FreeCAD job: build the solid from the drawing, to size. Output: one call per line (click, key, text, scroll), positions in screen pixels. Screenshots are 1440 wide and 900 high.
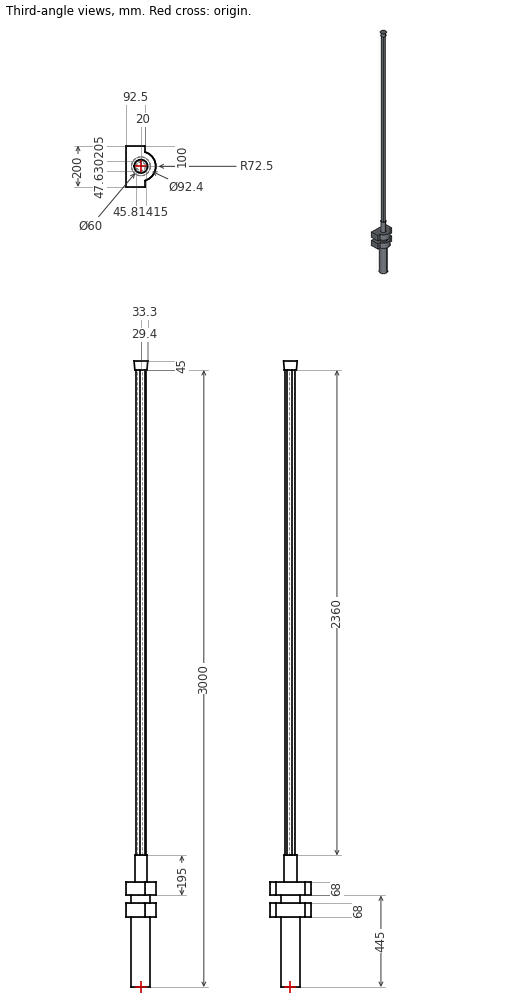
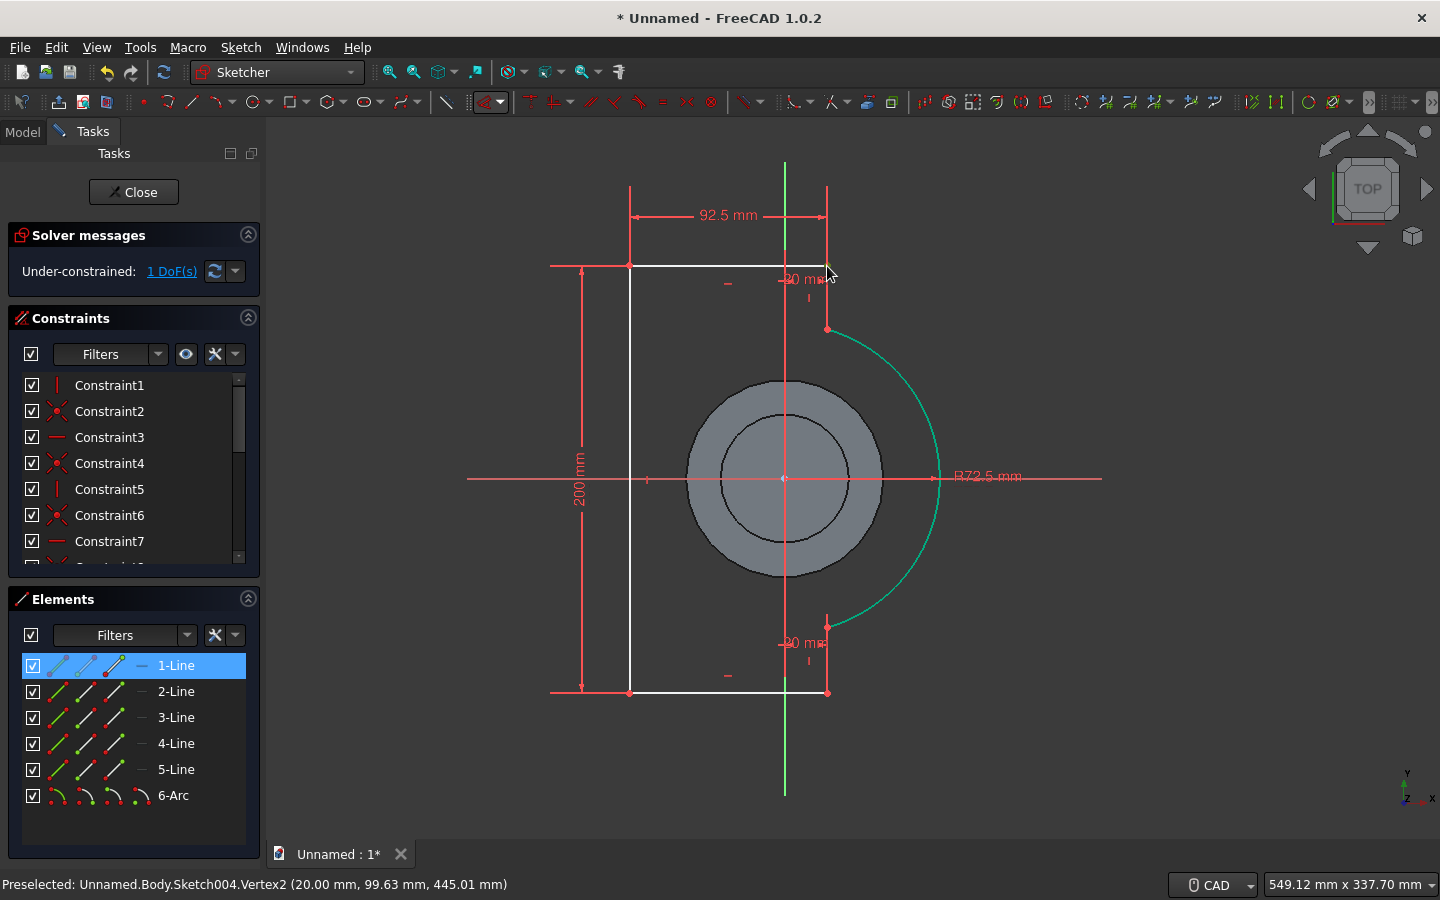
key(i)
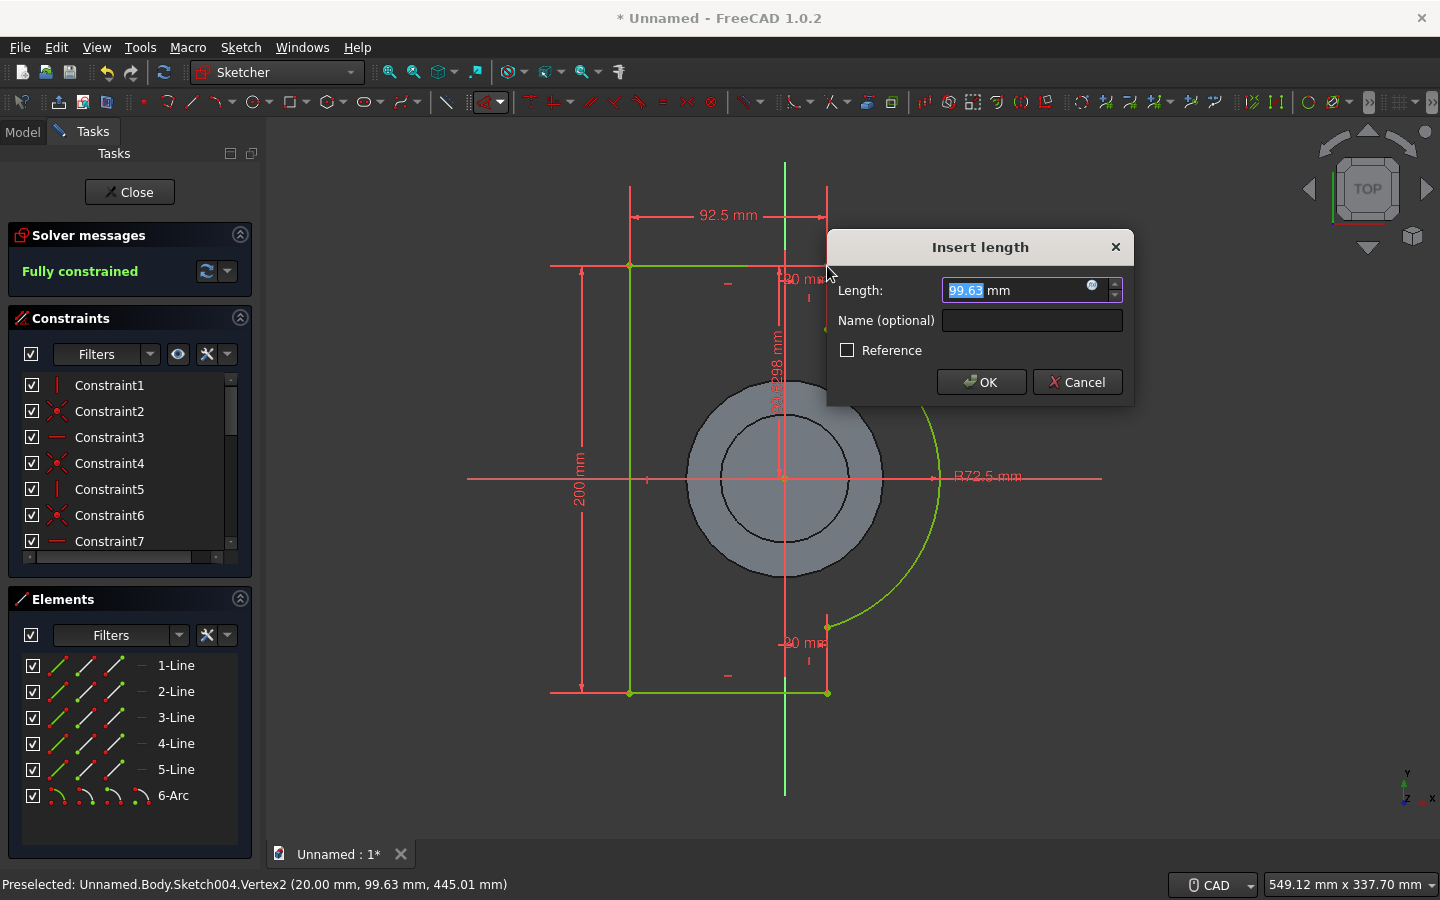
text(100)
key(Return)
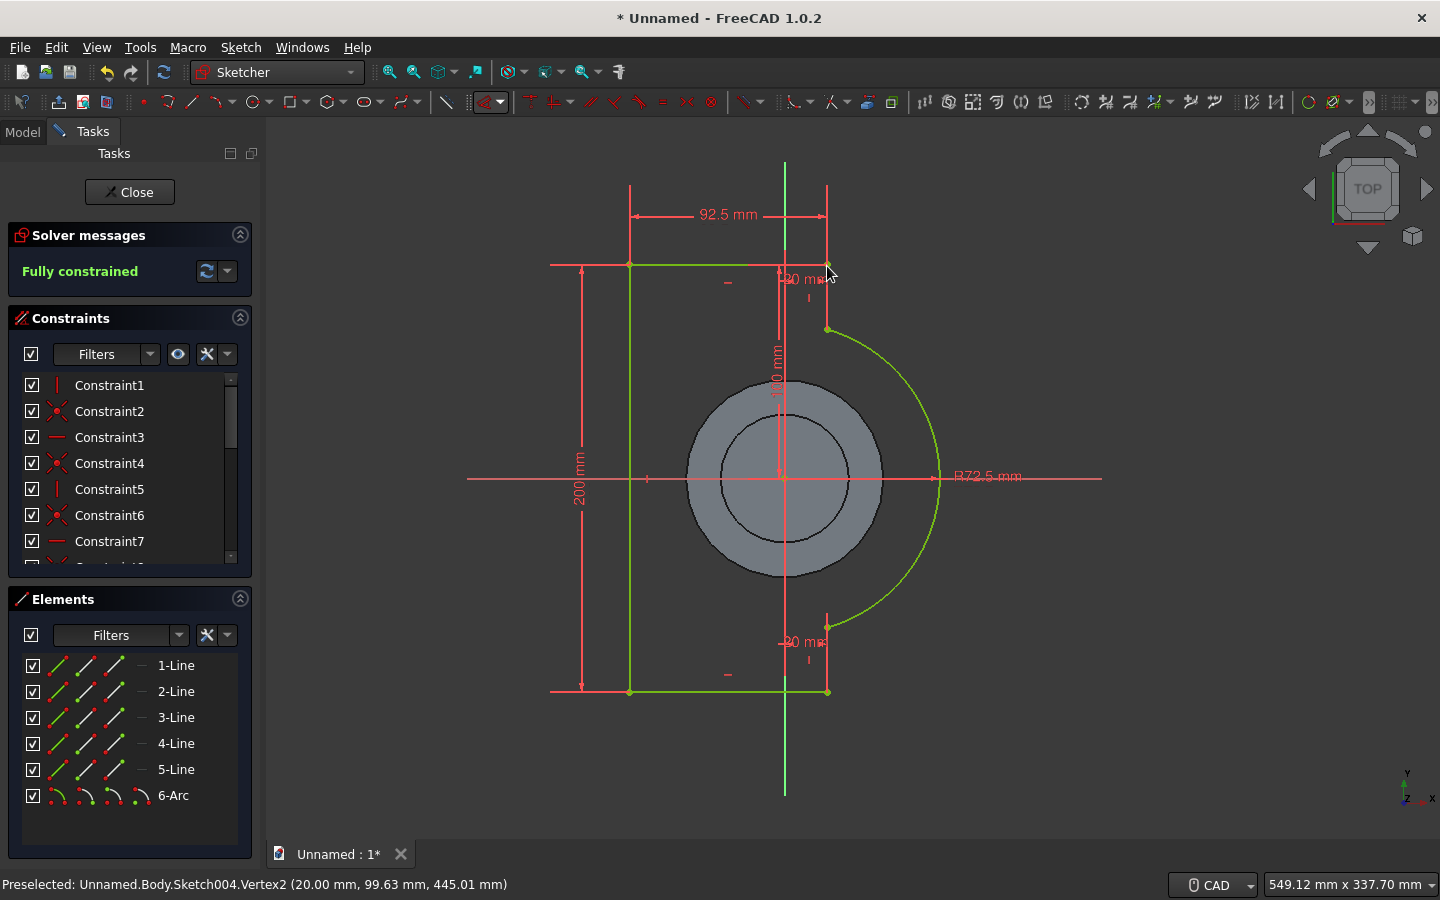
click(130, 192)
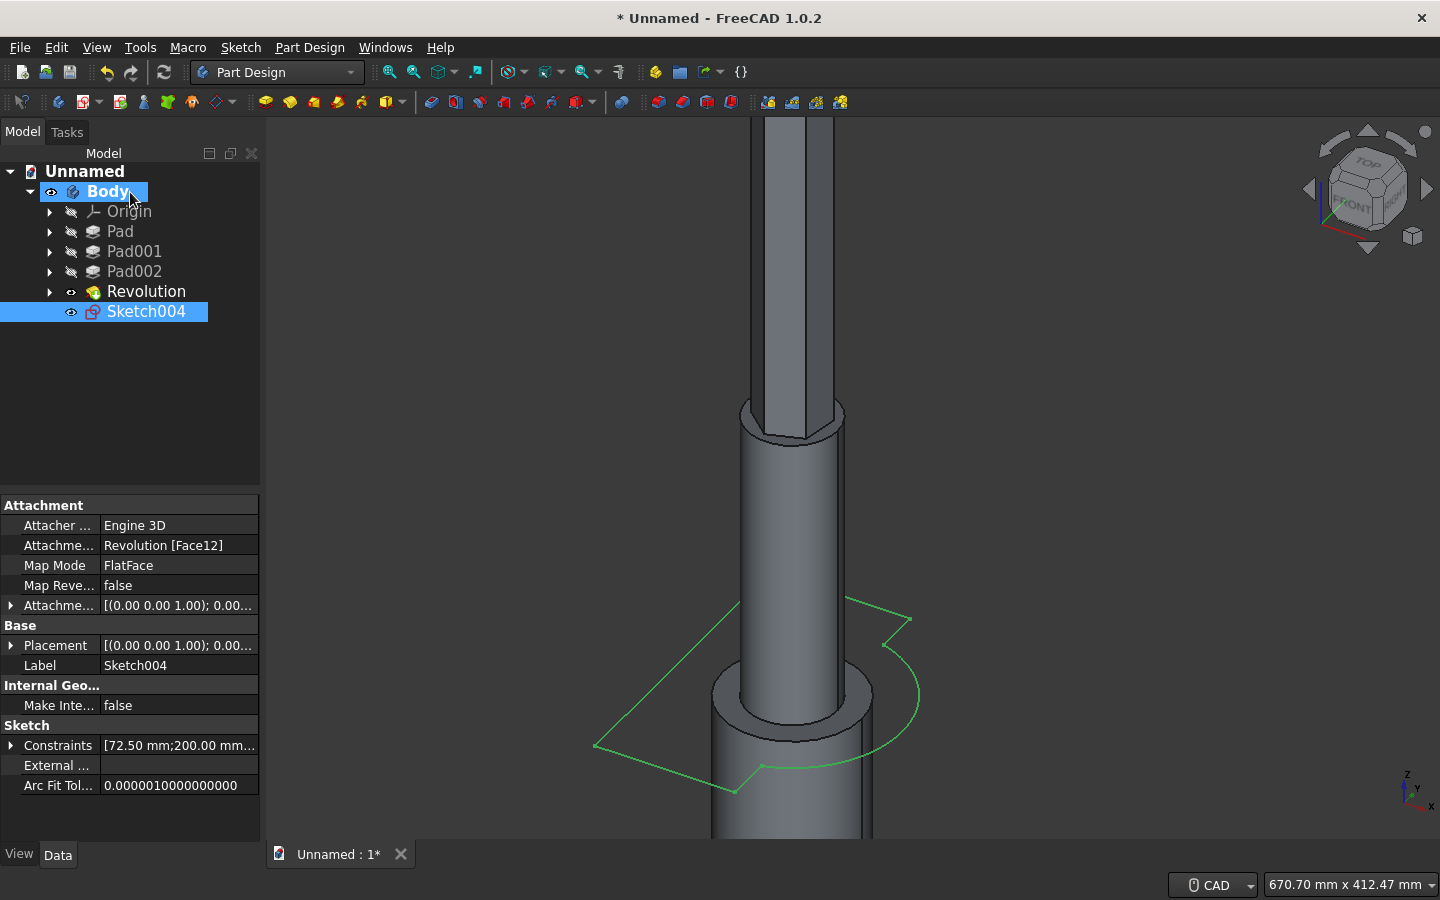
click(266, 102)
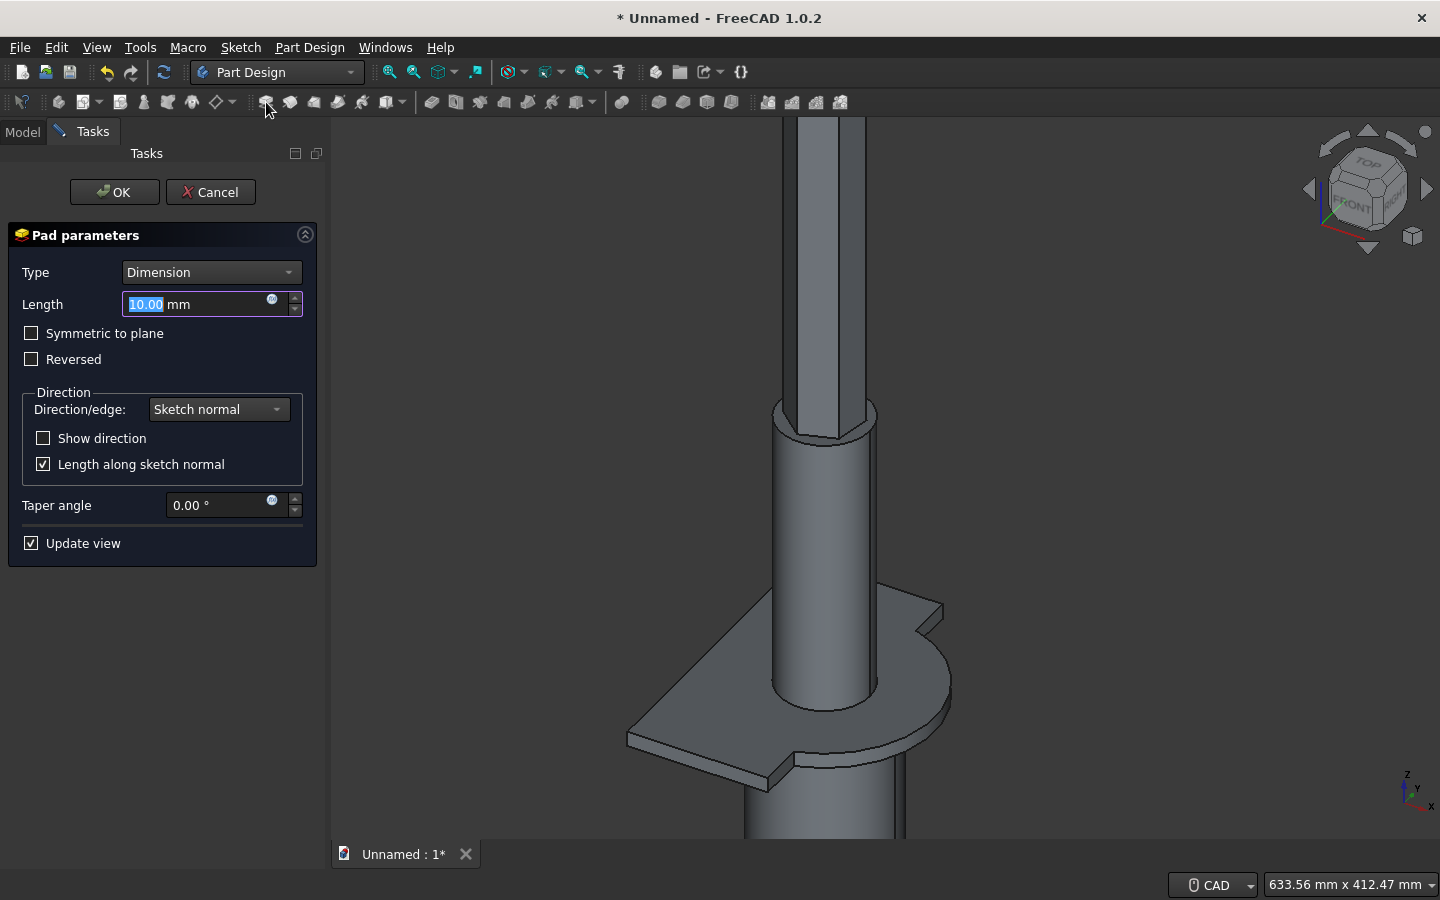
text(68)
key(Tab)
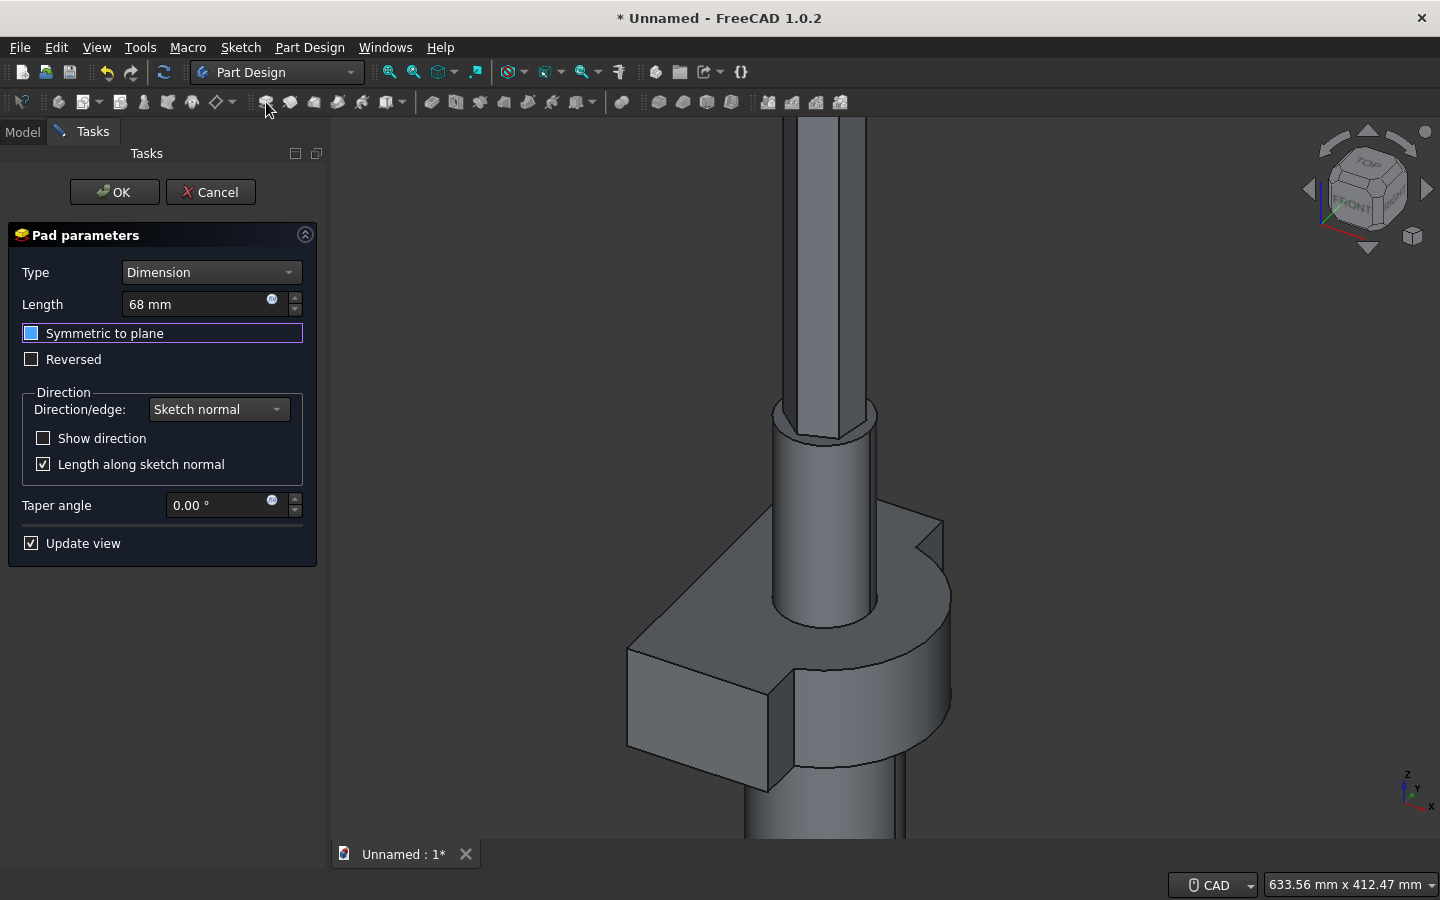
click(115, 192)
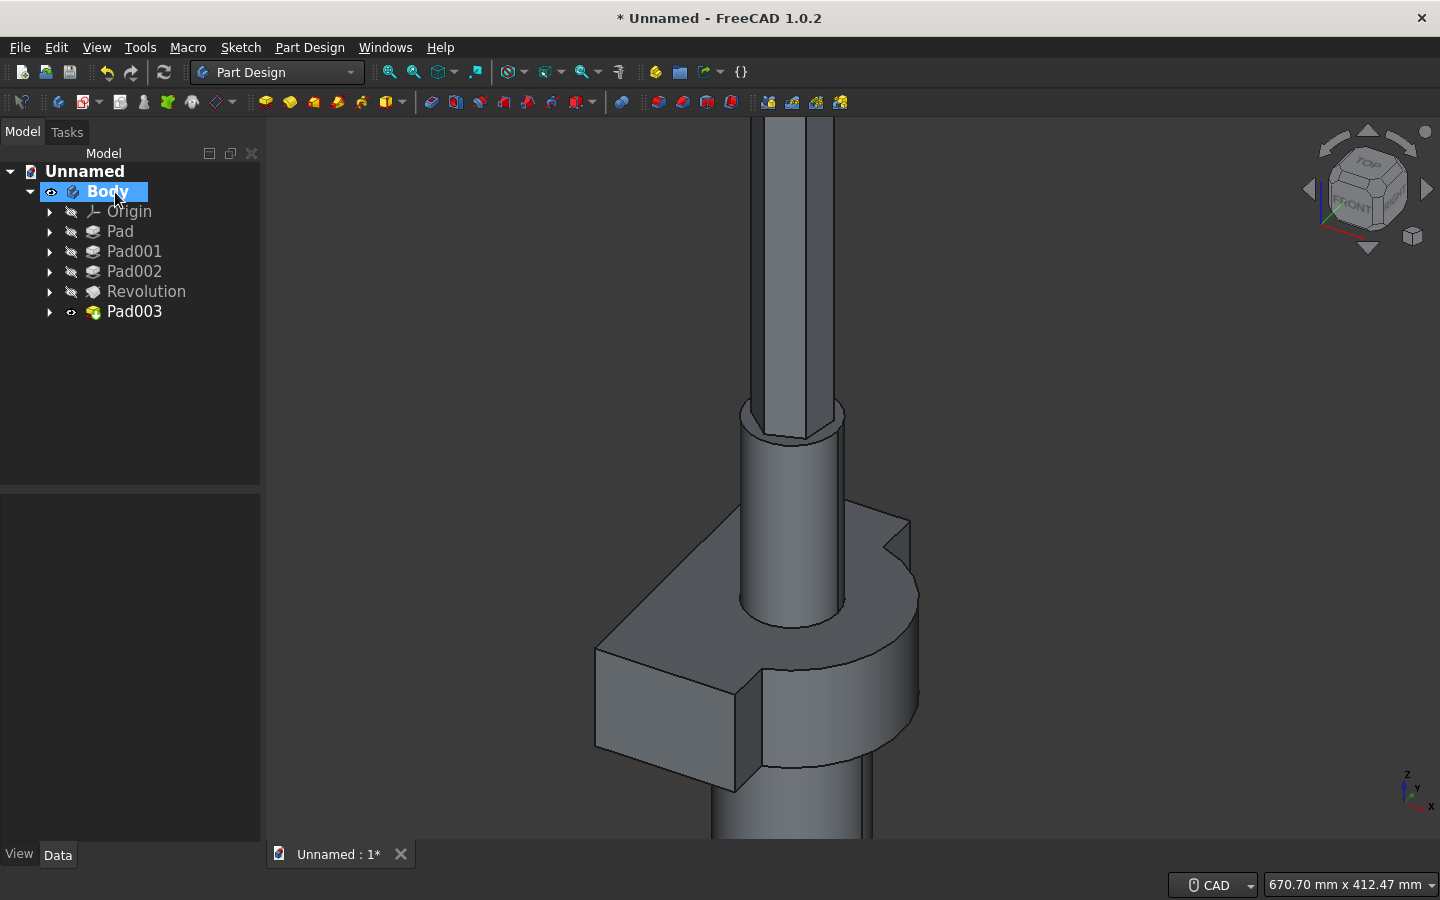
key(v)
key(f)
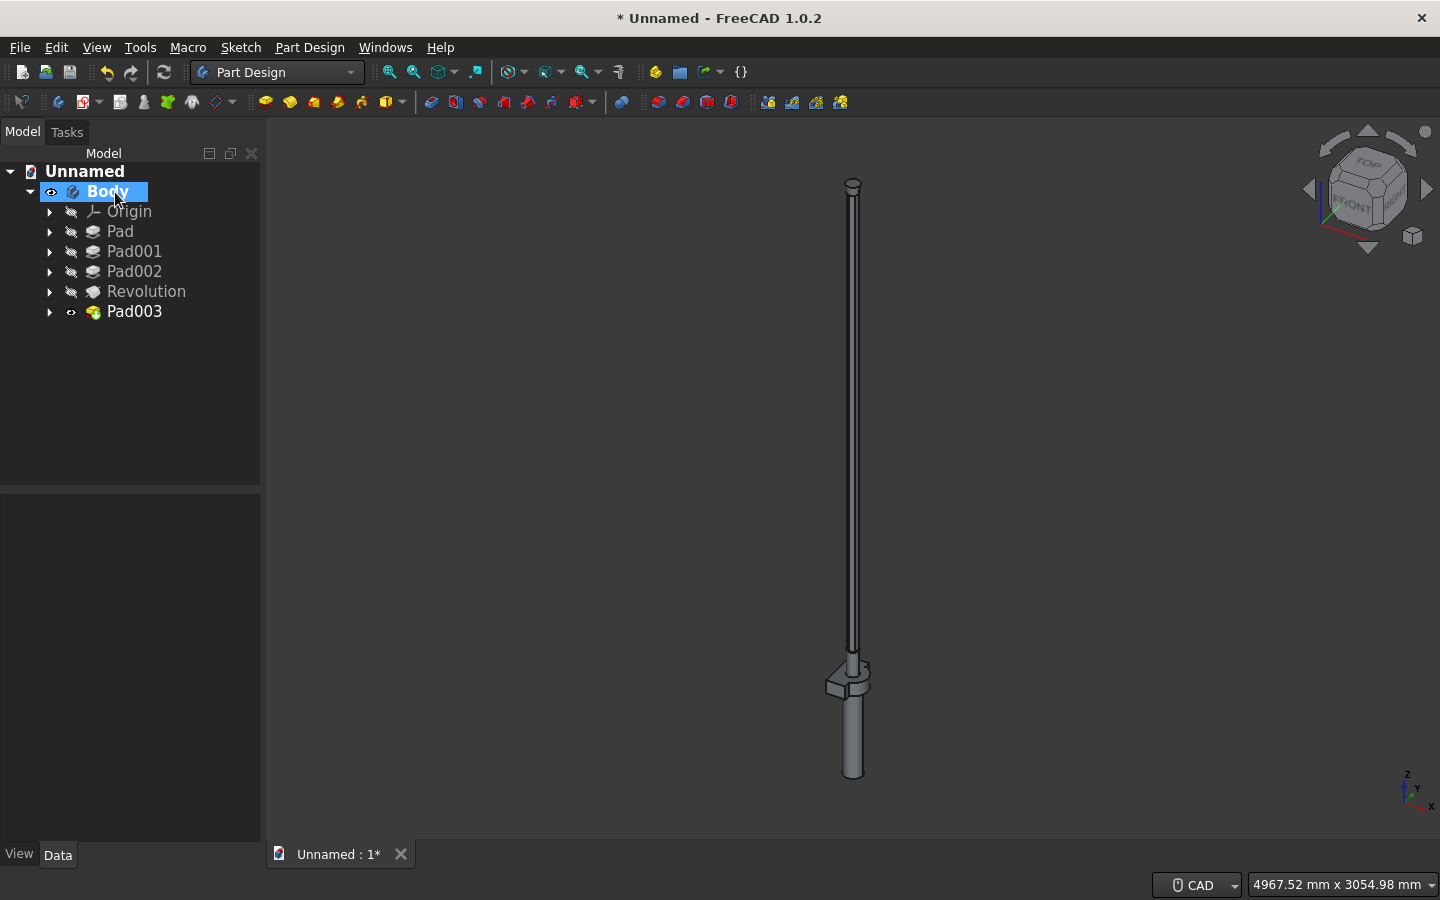
click(50, 212)